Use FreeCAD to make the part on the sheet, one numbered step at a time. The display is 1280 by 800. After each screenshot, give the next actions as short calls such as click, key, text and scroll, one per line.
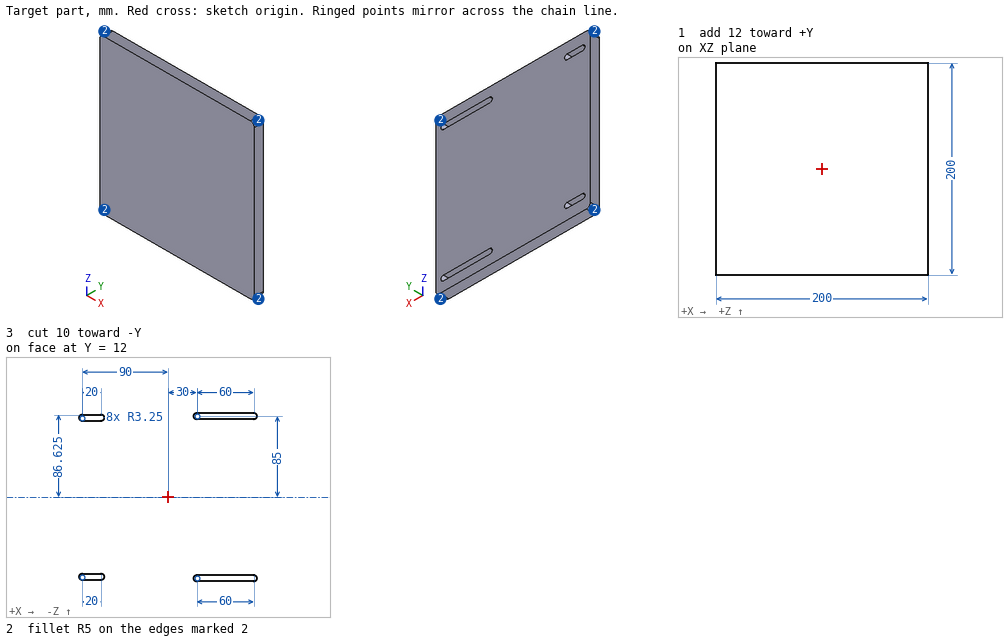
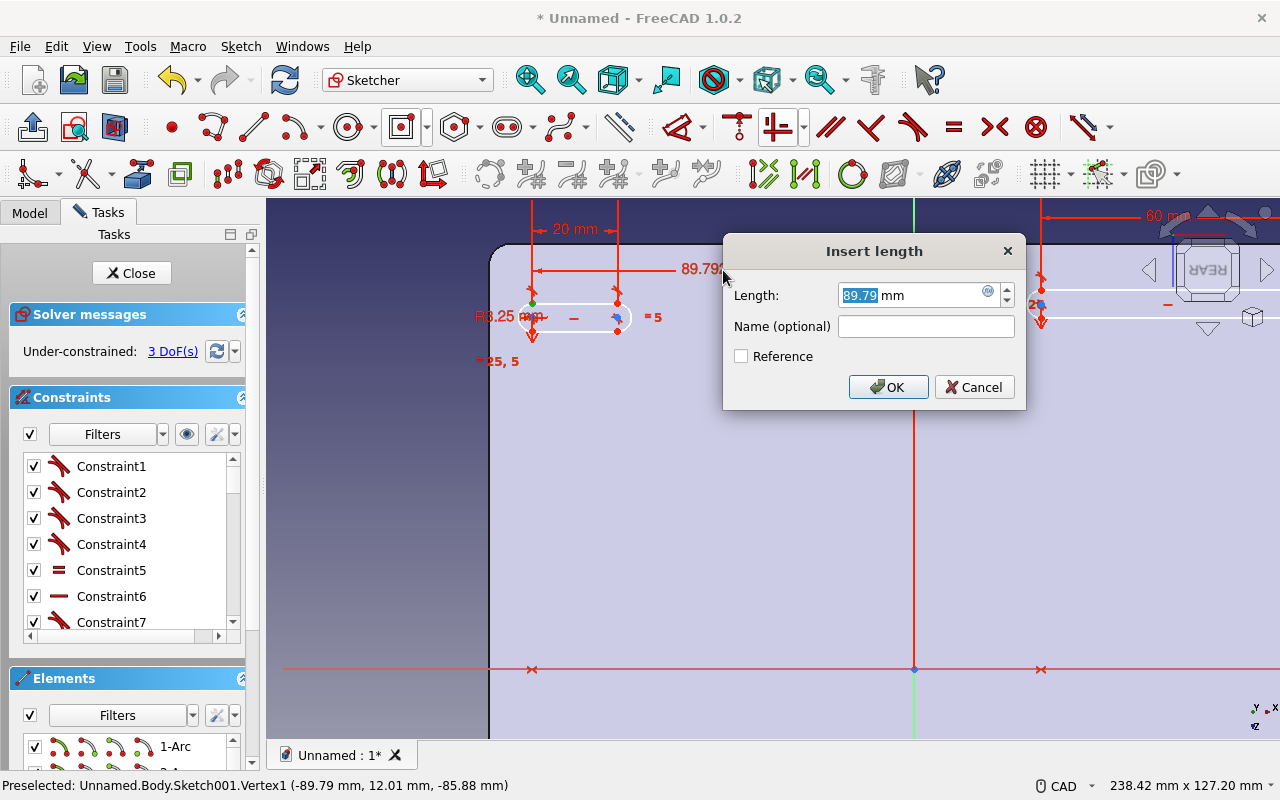
text(90)
key(Return)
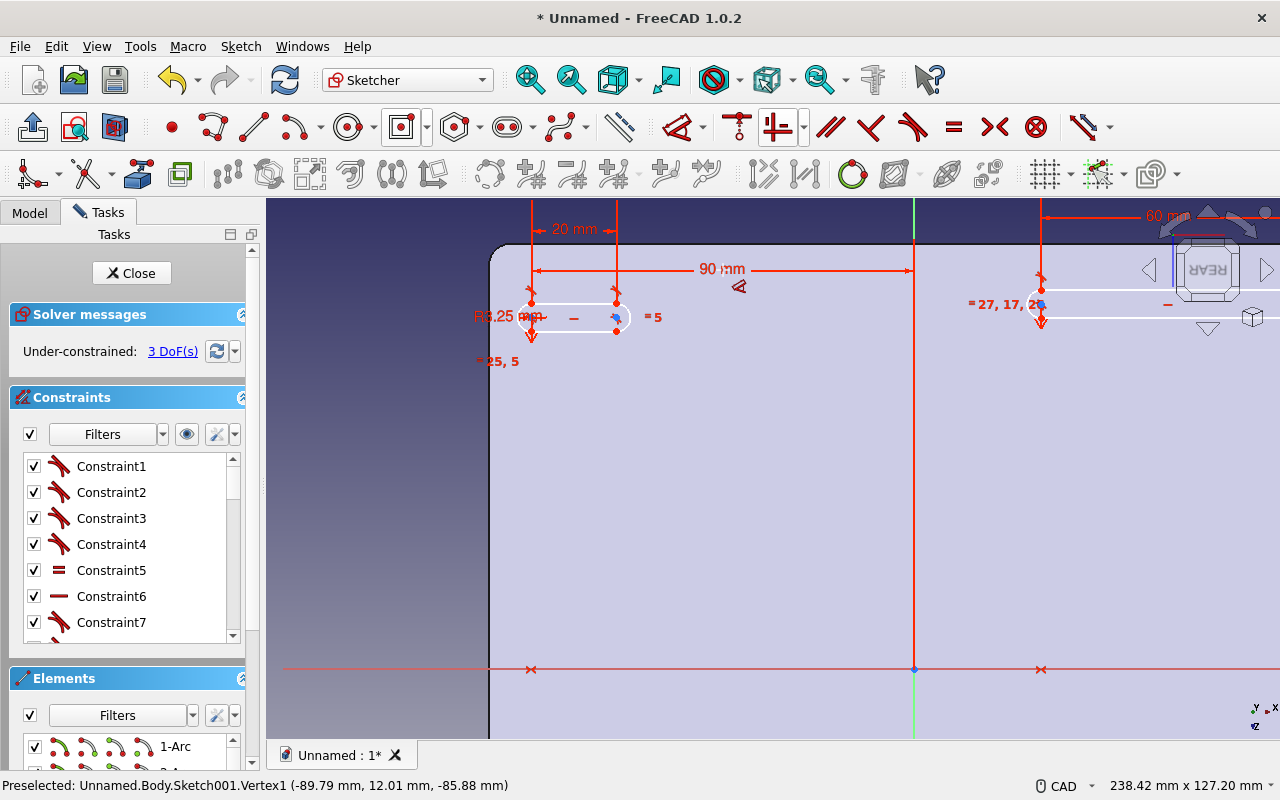
click(1041, 290)
click(978, 256)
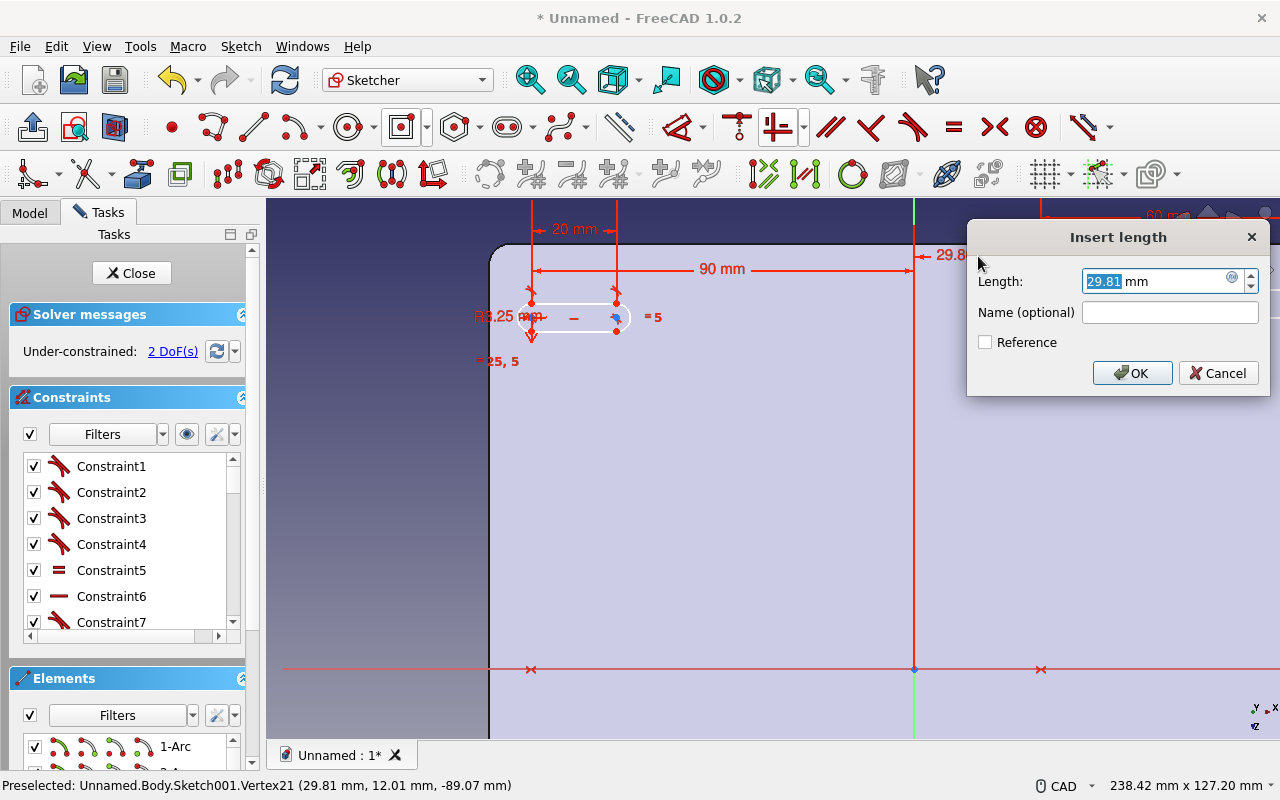
text(30)
key(Return)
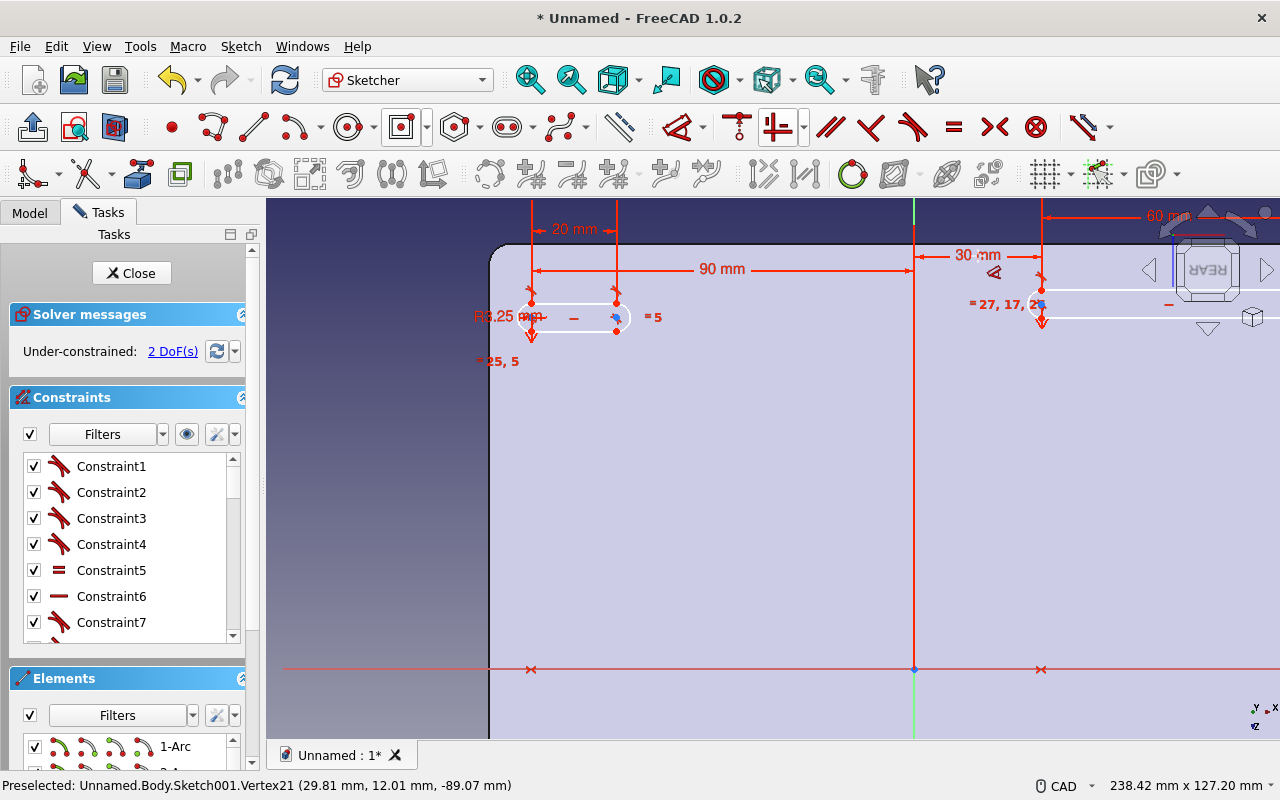
click(1042, 304)
click(1076, 487)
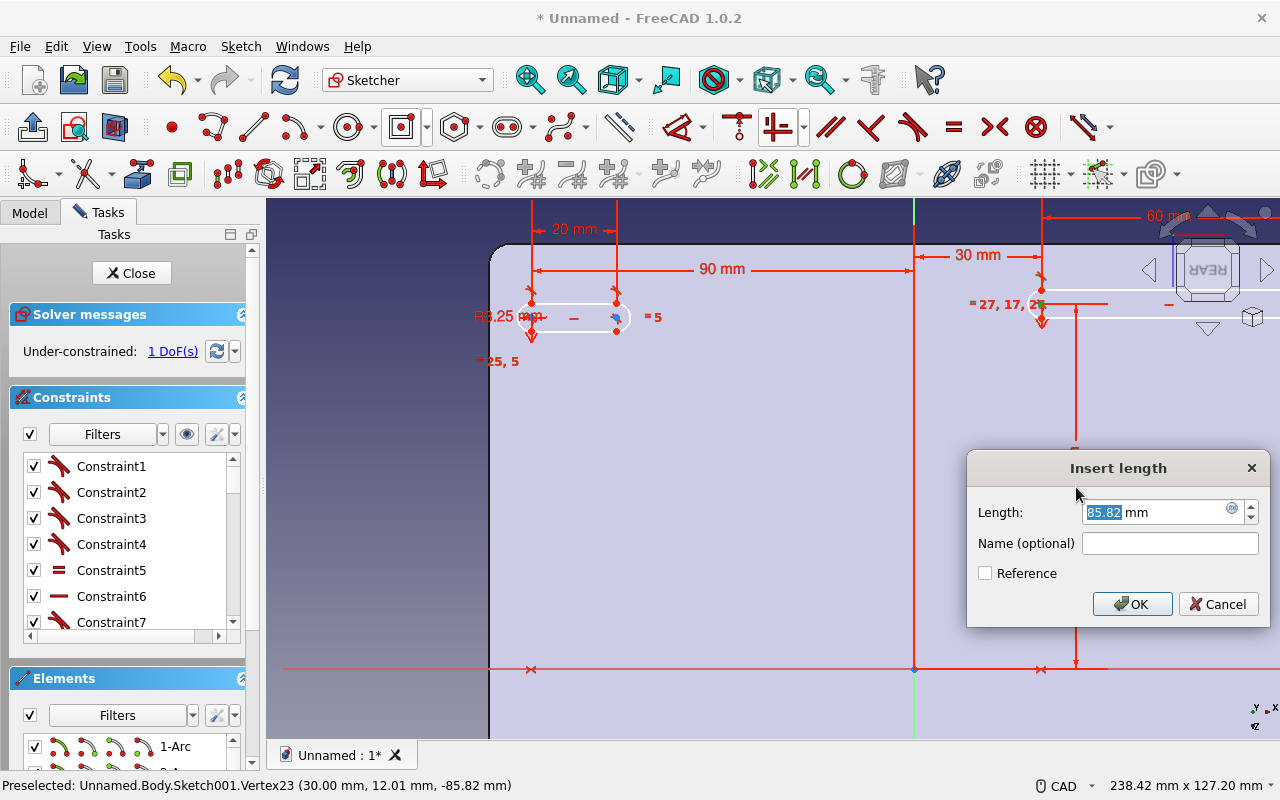
text(85)
key(Return)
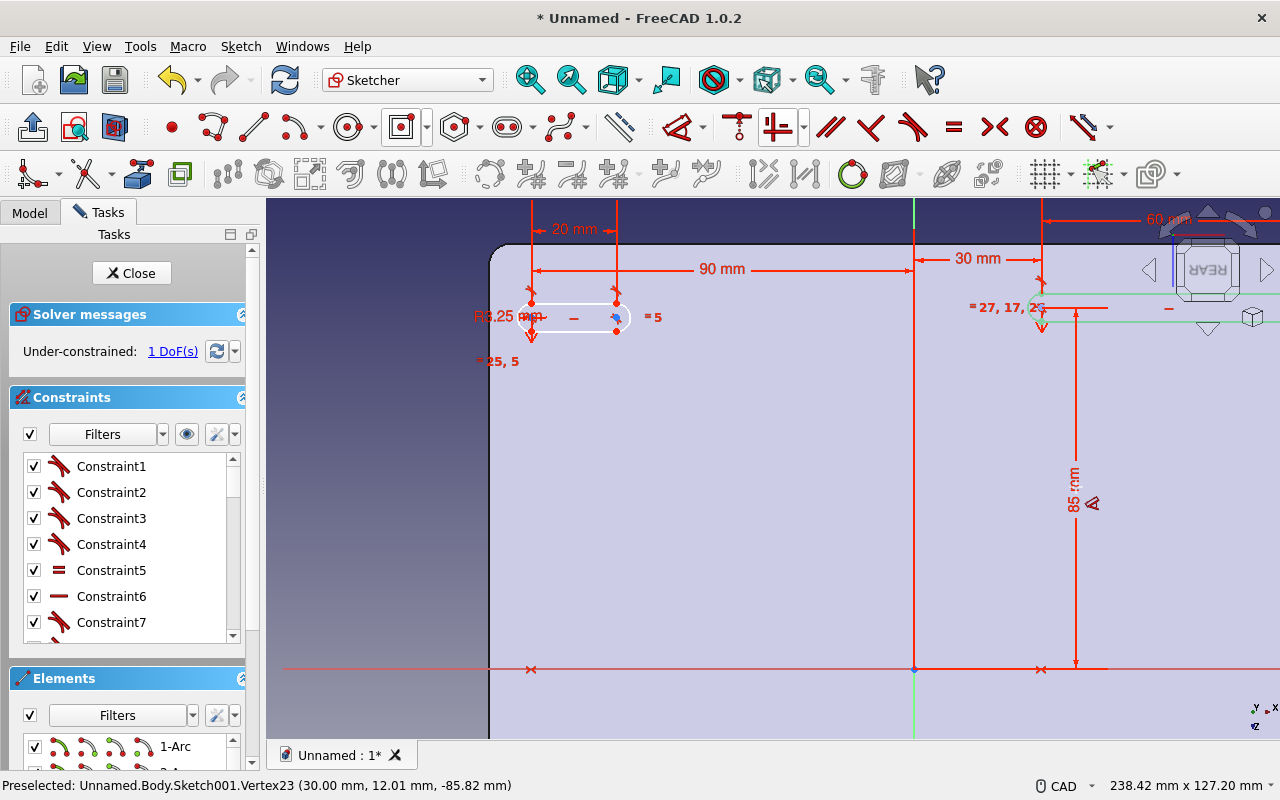
click(532, 304)
click(498, 487)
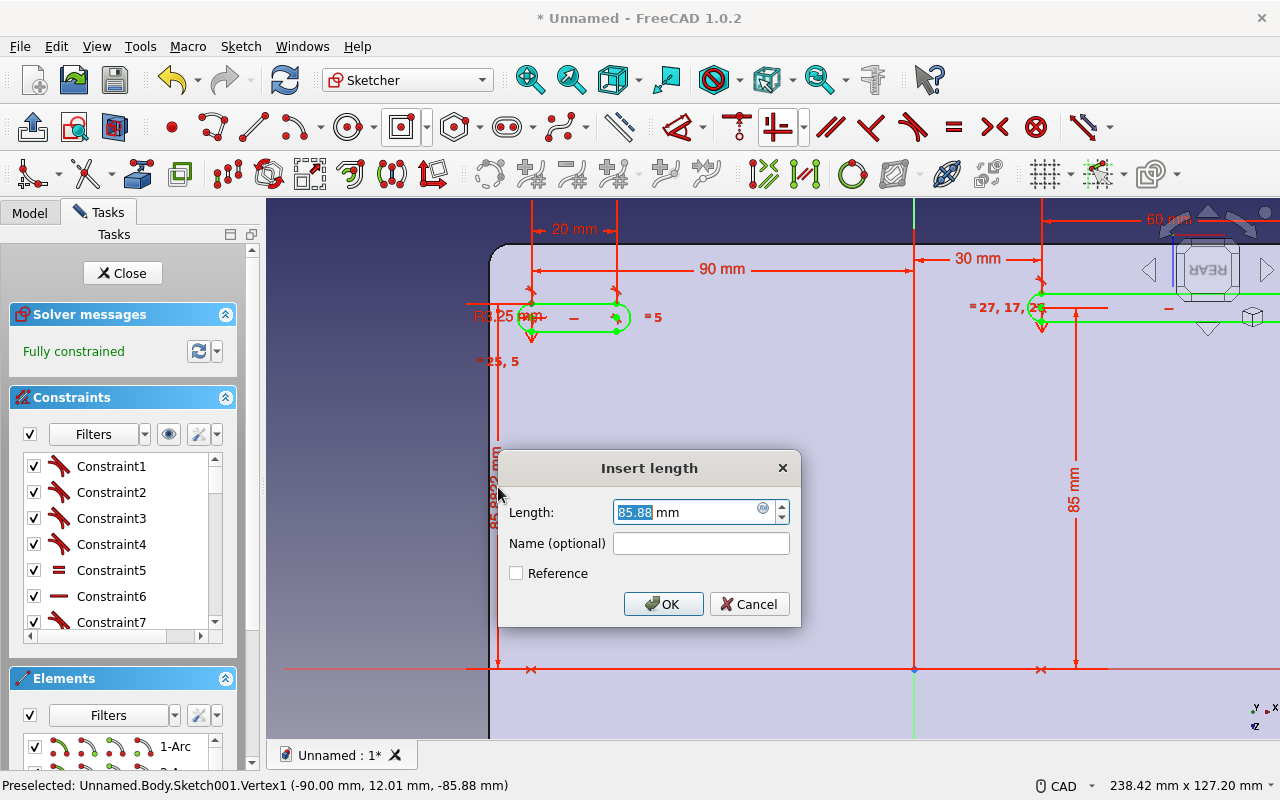
text(86.625)
key(Return)
key(Escape)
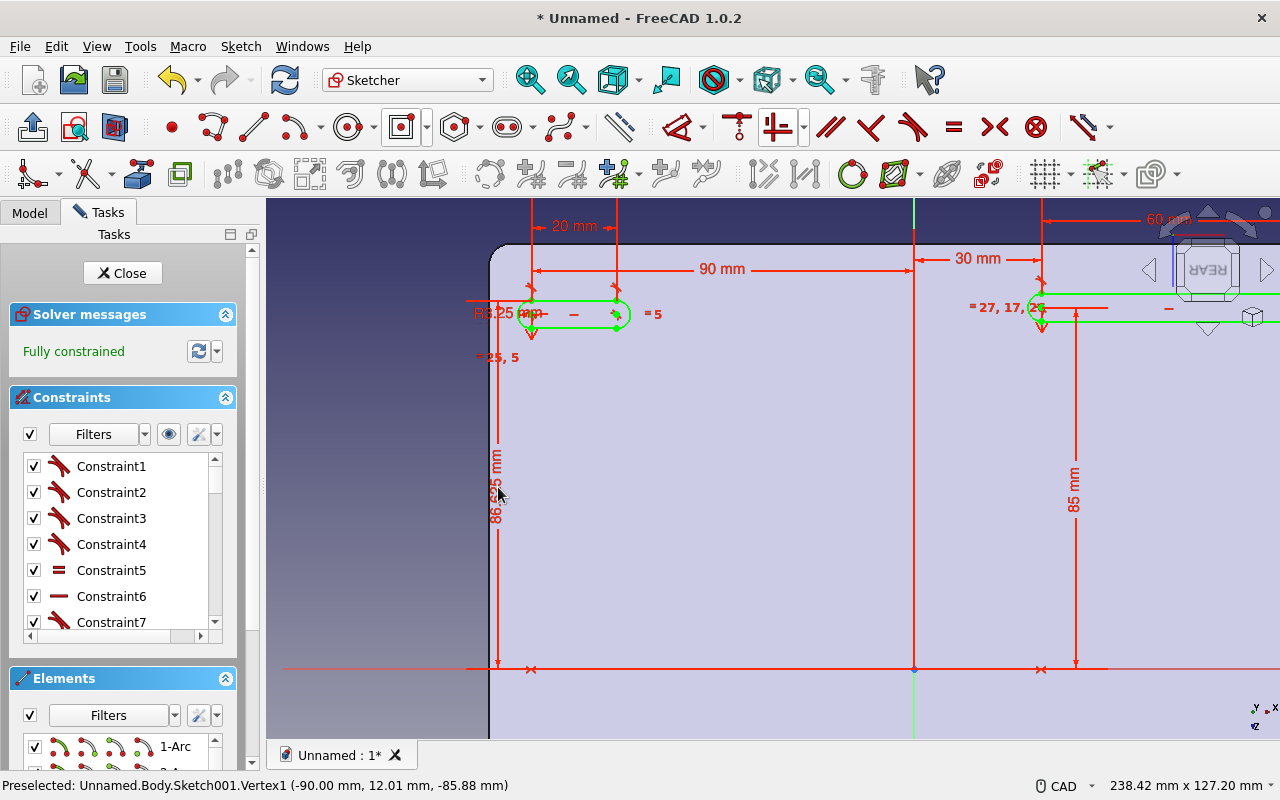
click(123, 273)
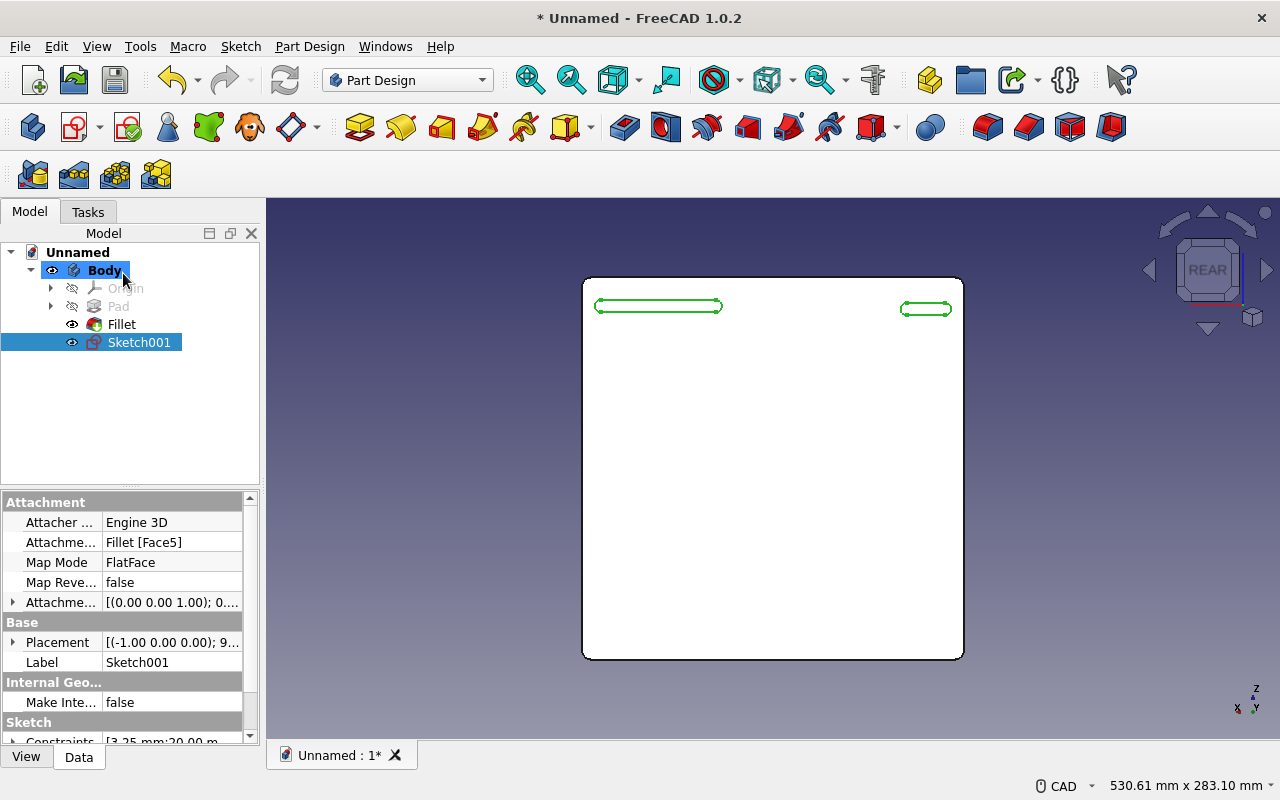
click(625, 128)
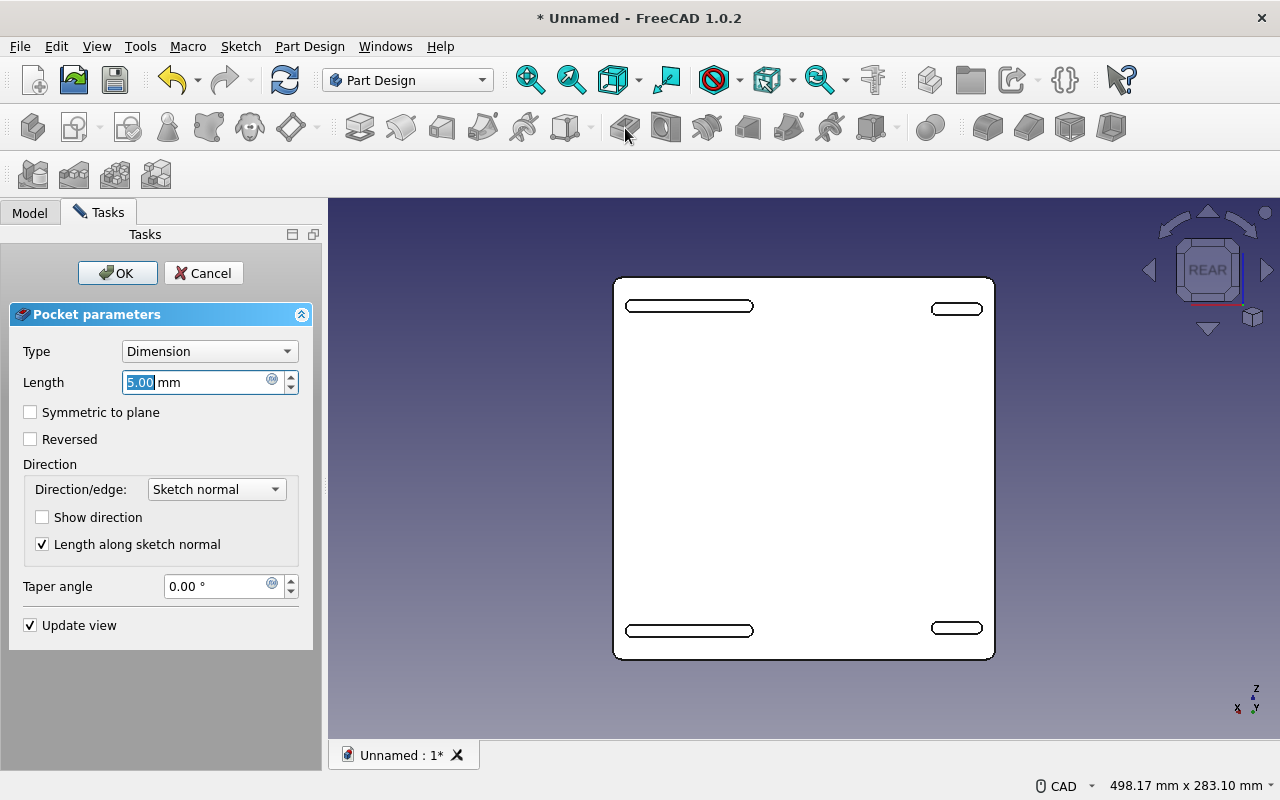
text(10)
key(Tab)